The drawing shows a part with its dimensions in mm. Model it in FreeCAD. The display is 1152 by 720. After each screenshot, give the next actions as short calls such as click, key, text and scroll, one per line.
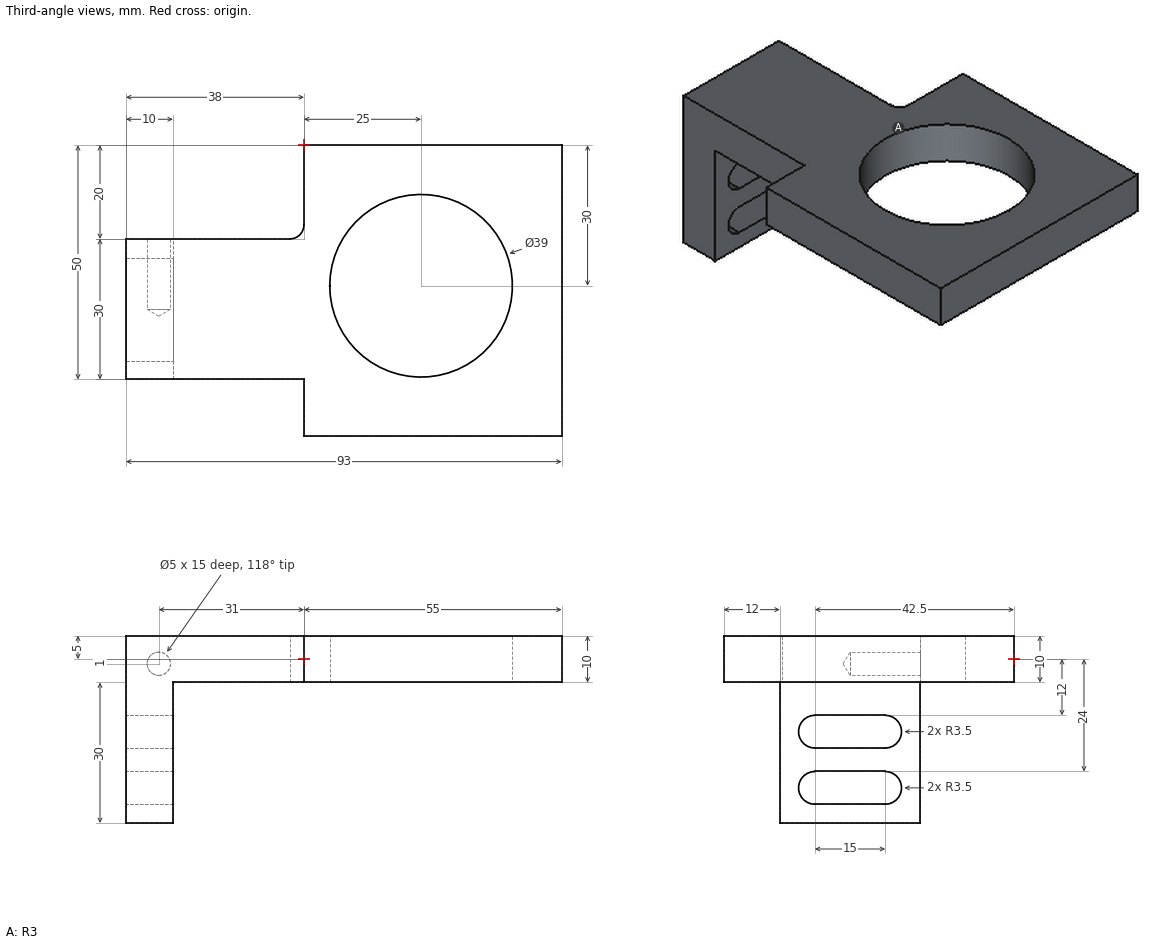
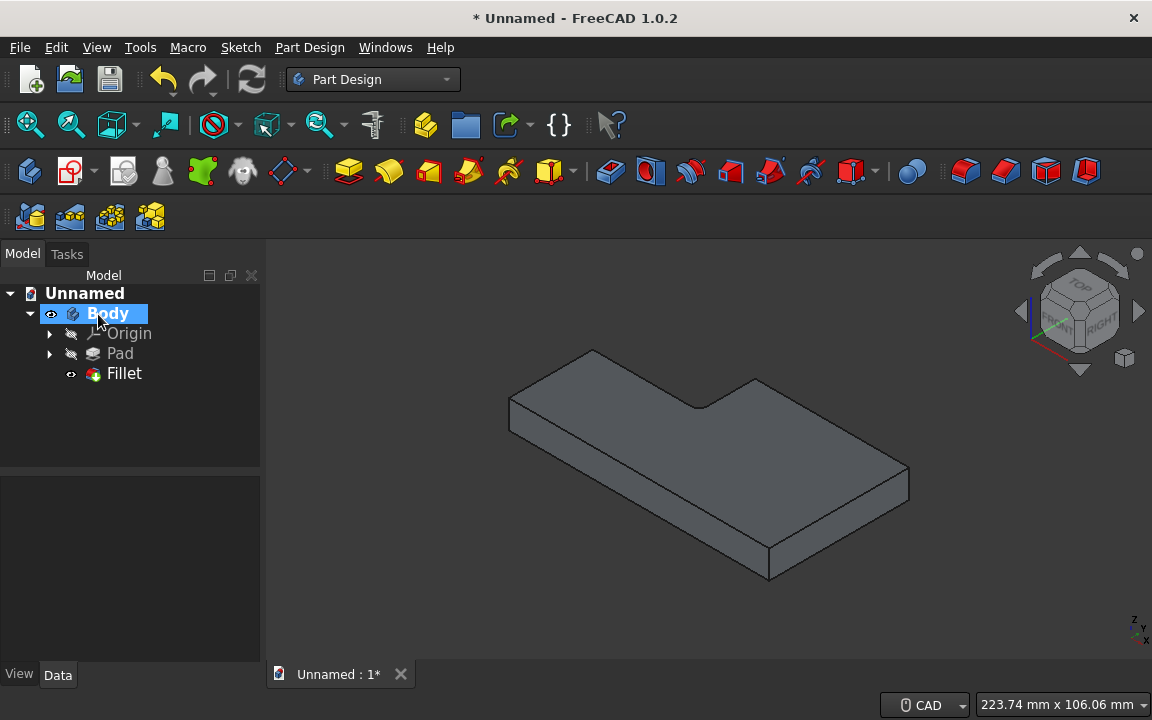
click(762, 448)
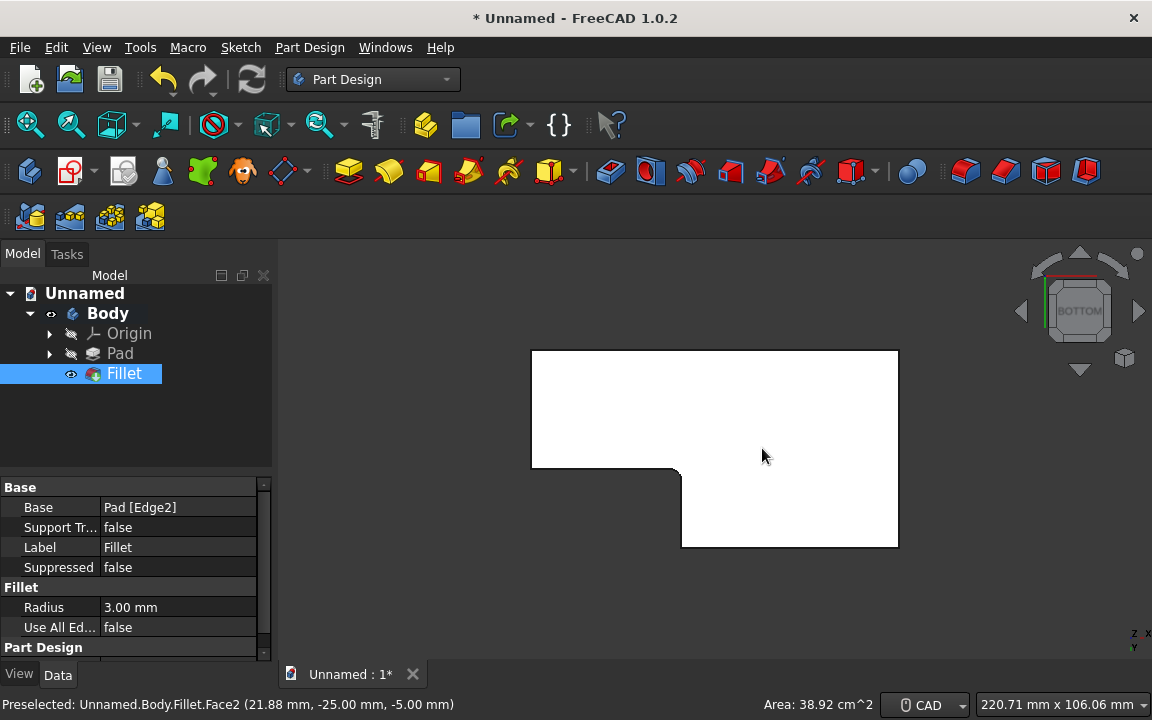
click(70, 172)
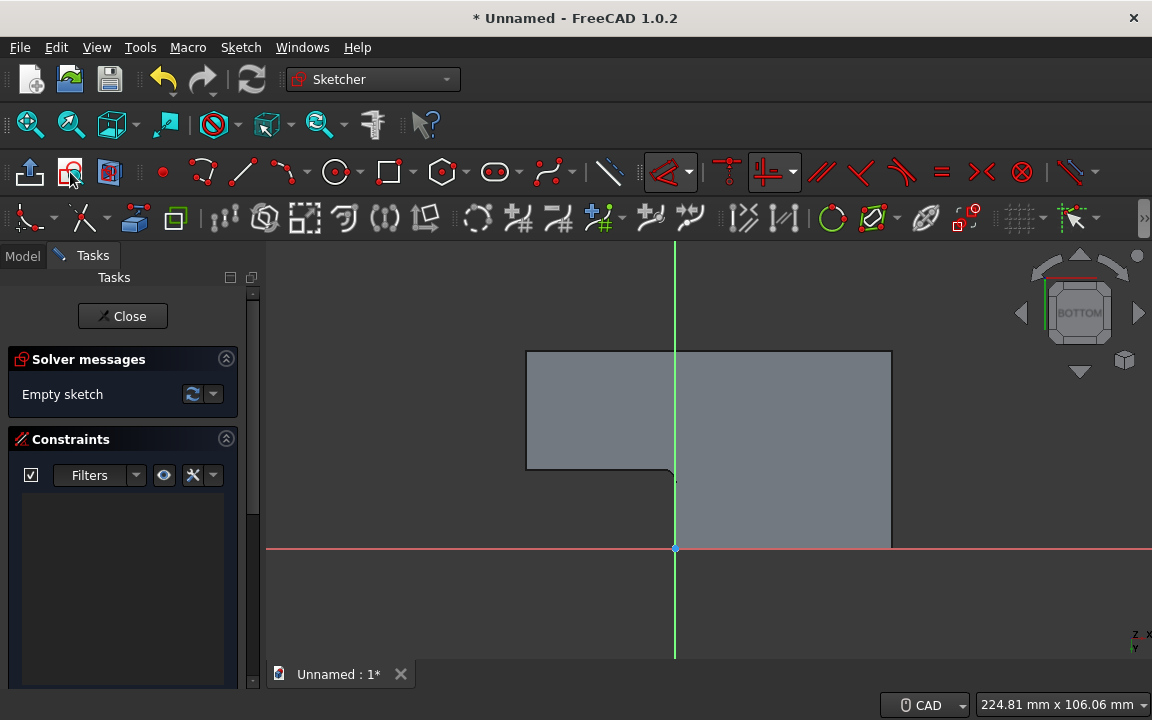
key(g)
key(c)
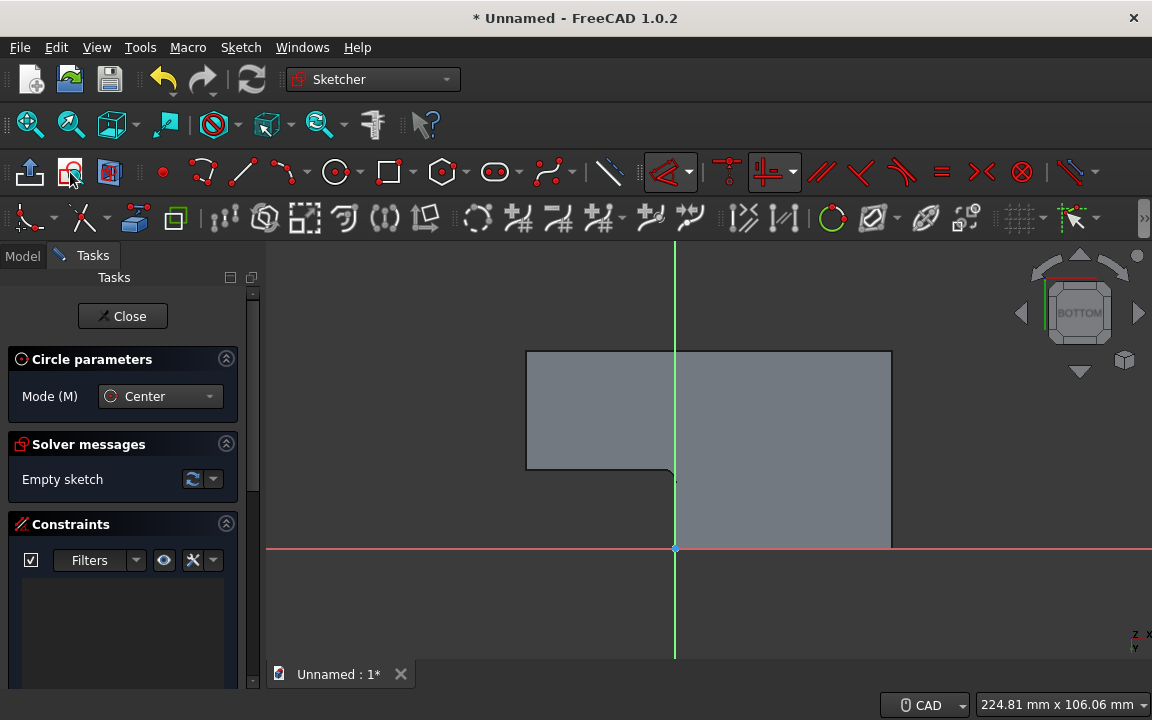
click(774, 430)
move(828, 376)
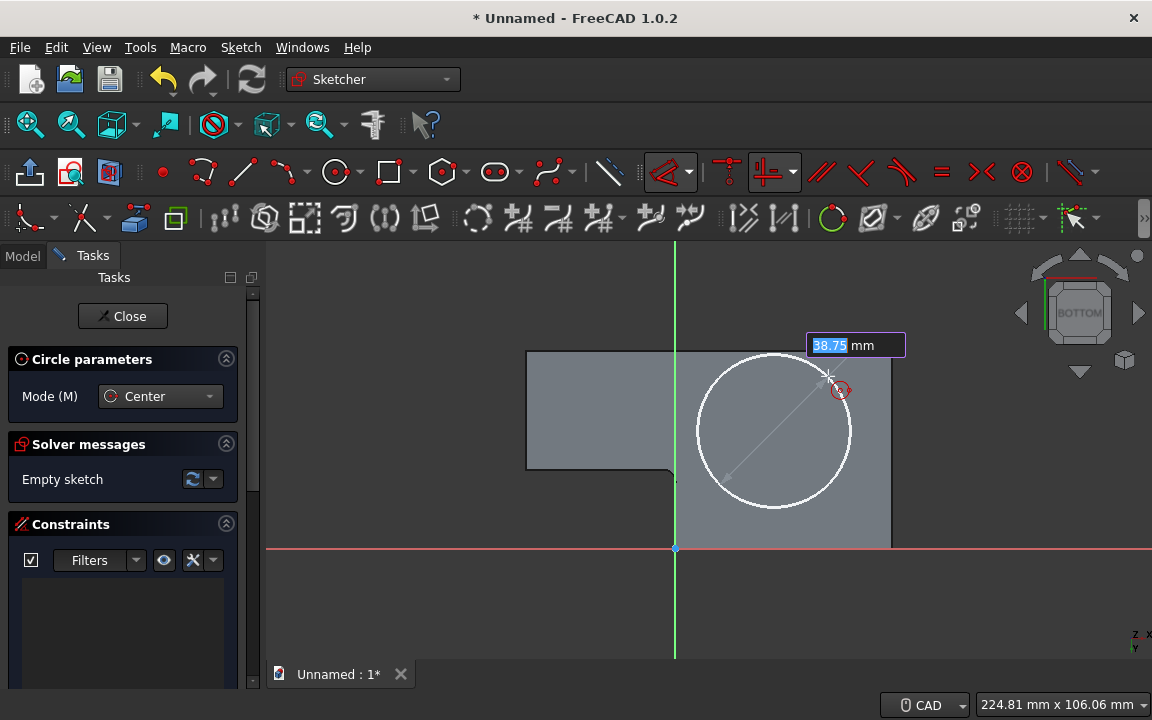
text(39)
key(Return)
key(Escape)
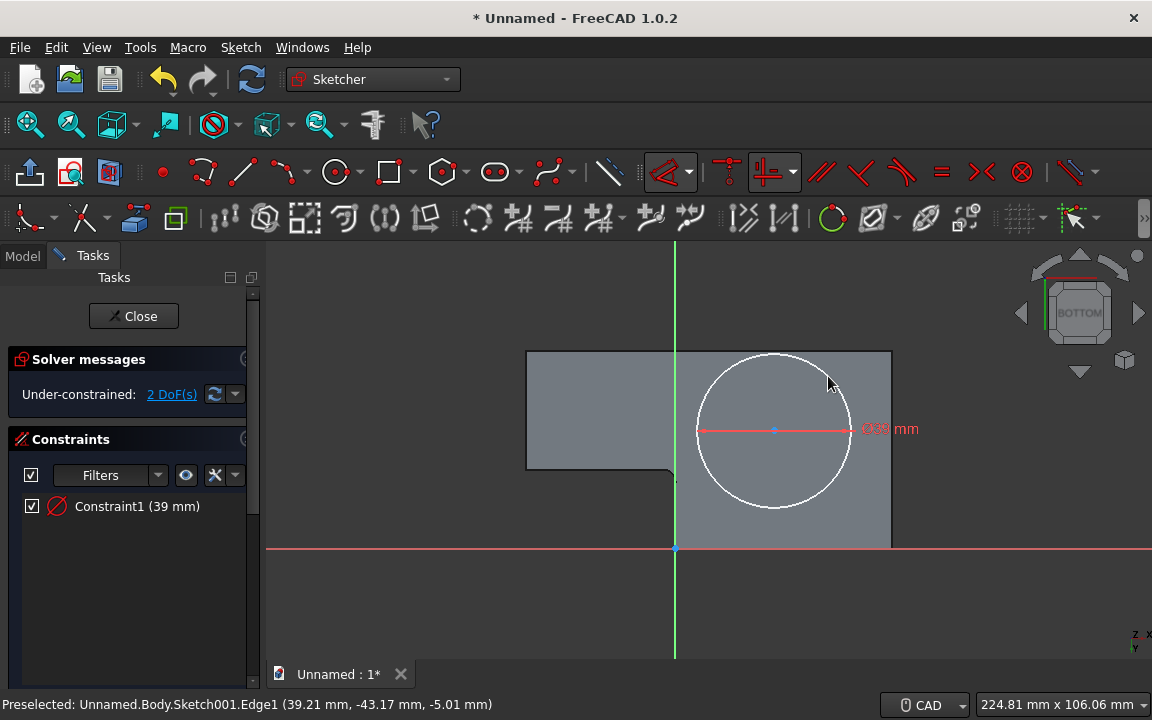
click(774, 431)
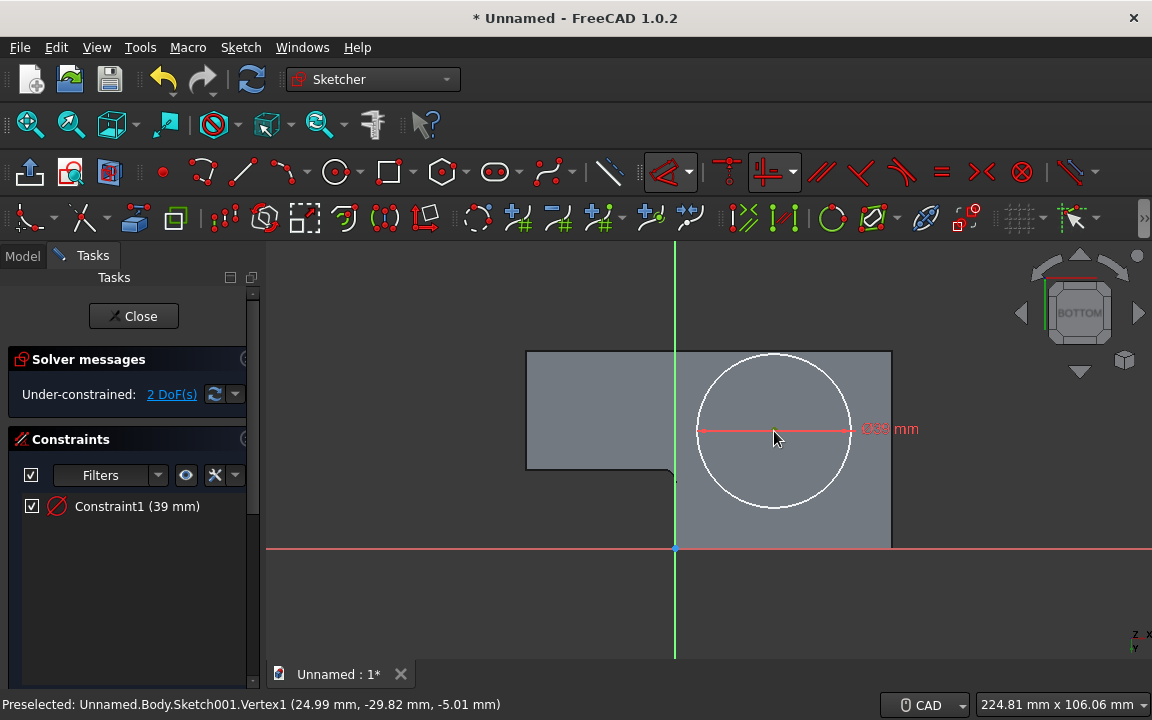
key(l)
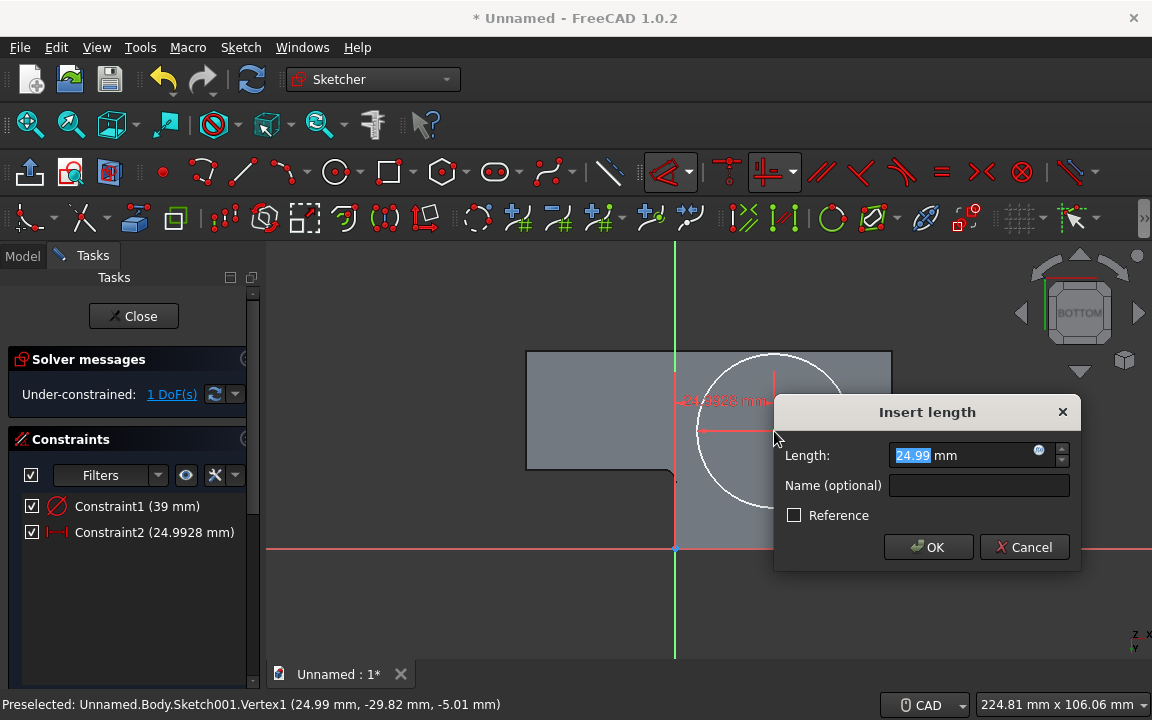
text(25)
key(Return)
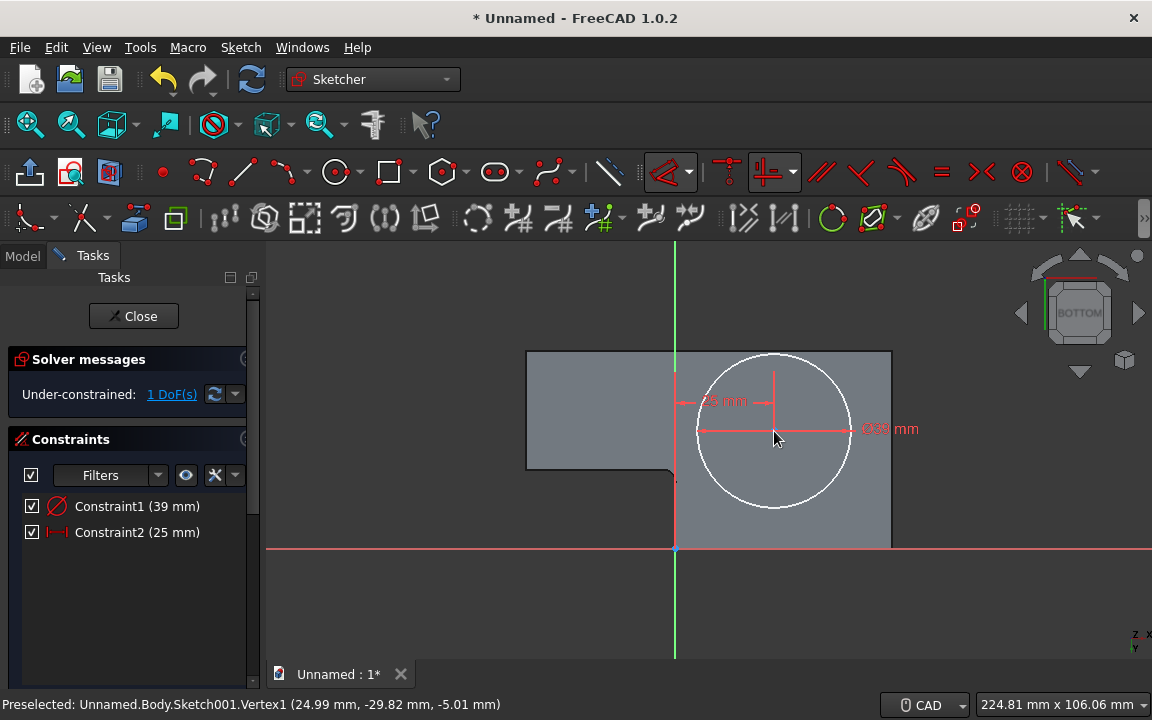
click(774, 431)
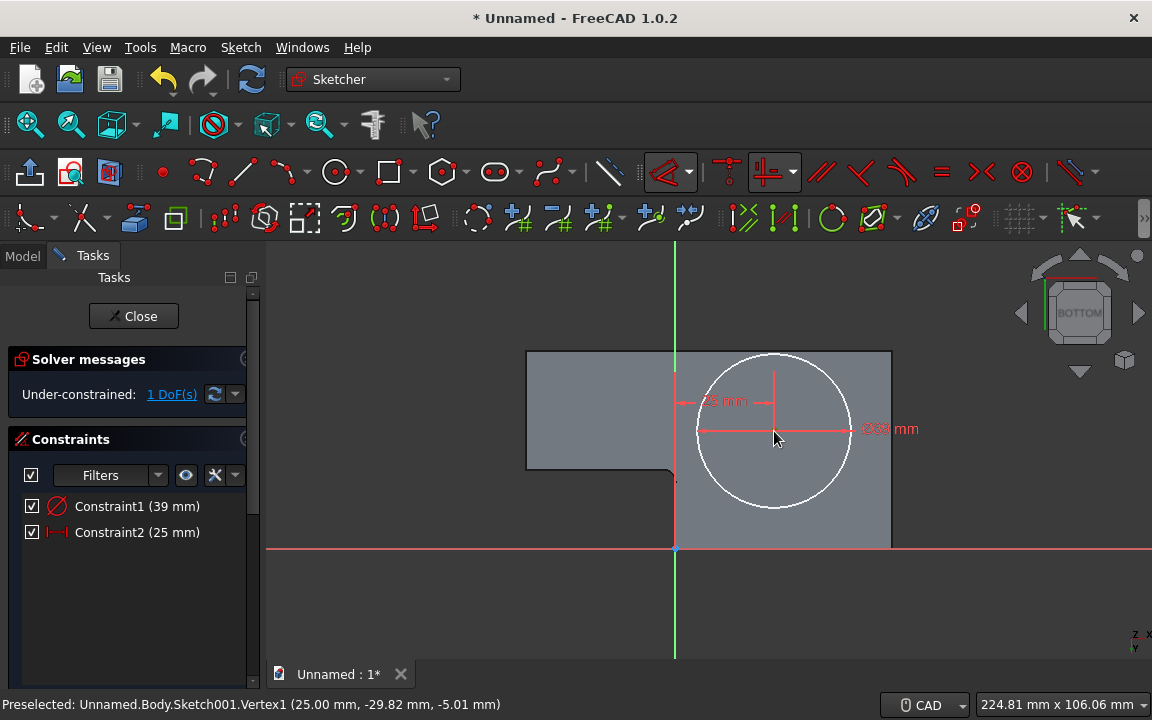
key(i)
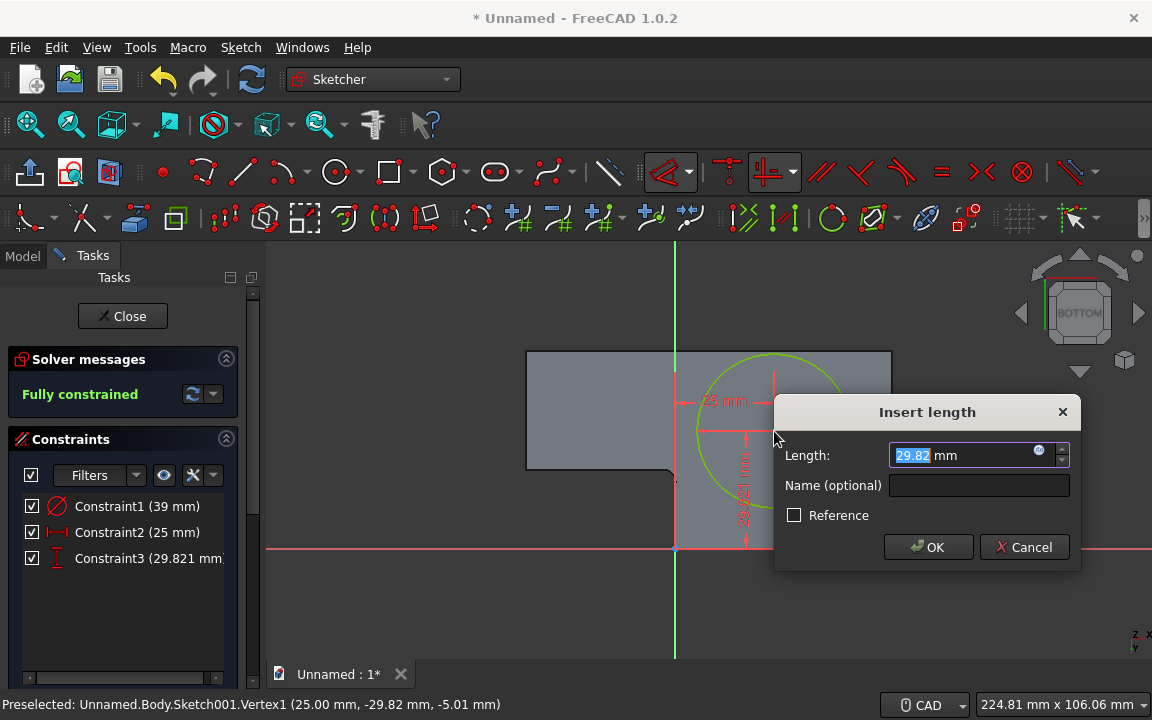
text(30)
key(Return)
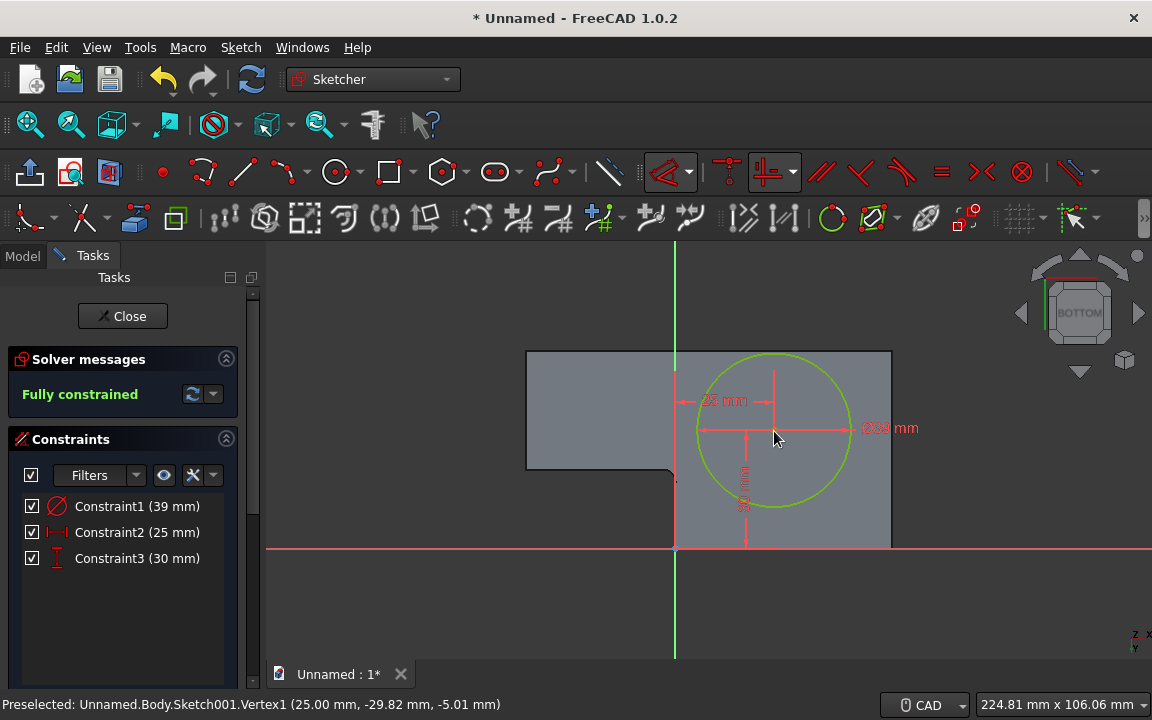
click(123, 316)